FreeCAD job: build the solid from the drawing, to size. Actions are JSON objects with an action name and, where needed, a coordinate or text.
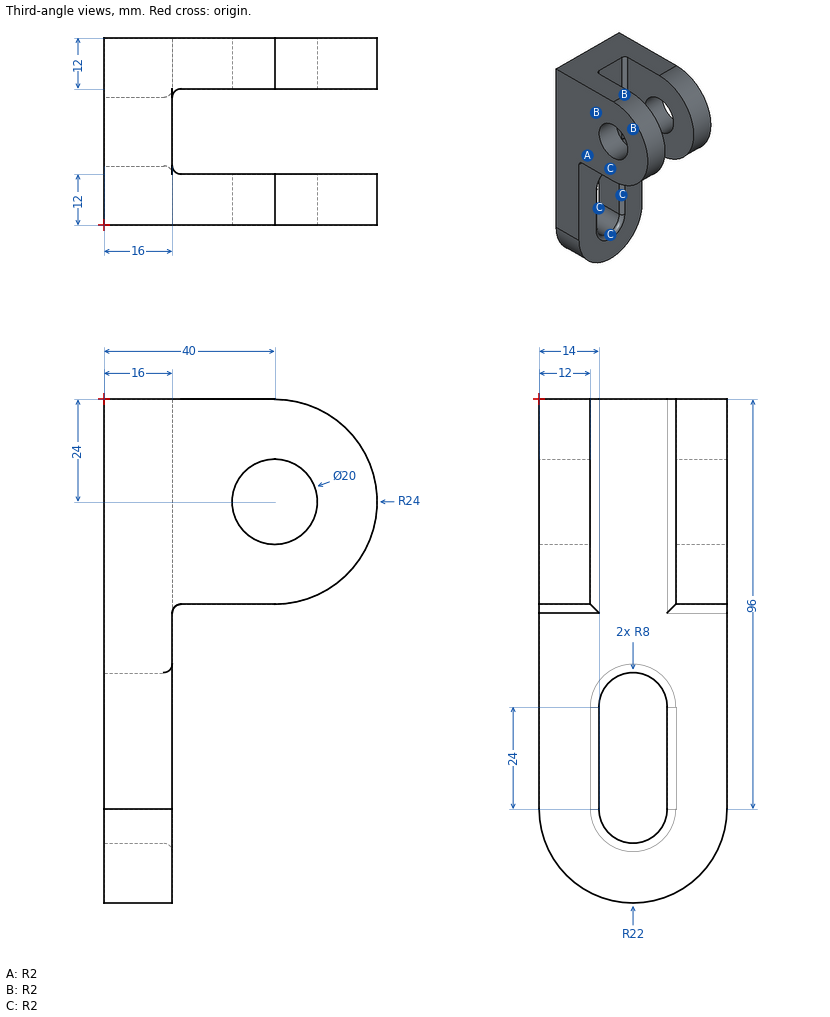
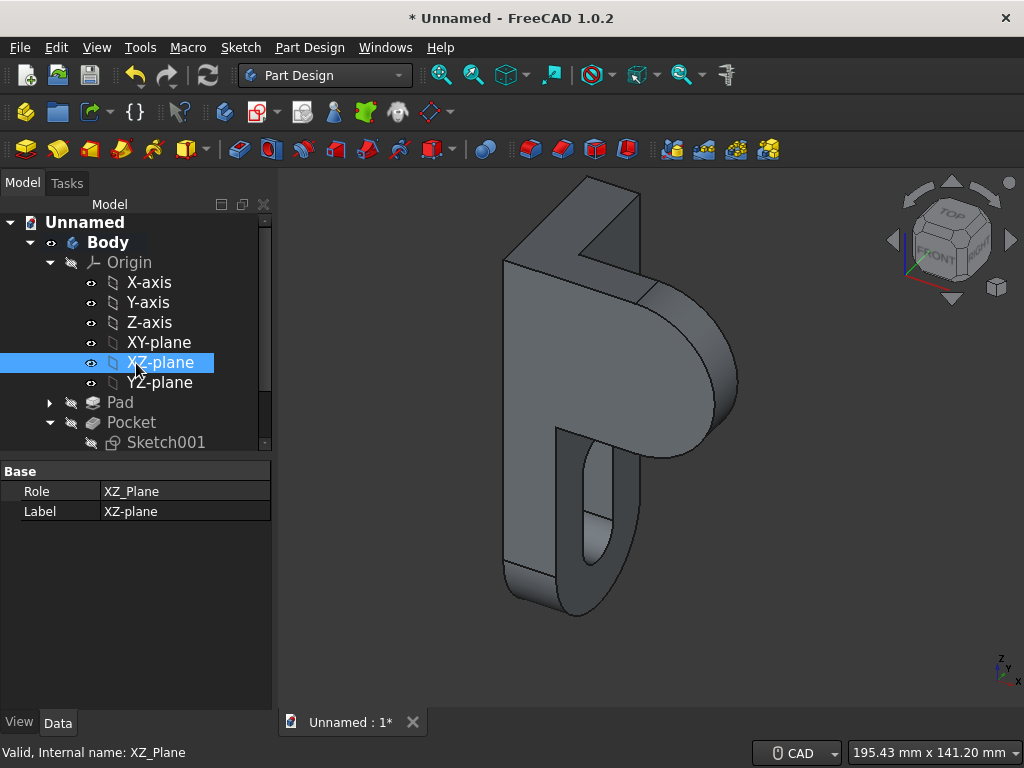
{"action": "left_click", "coordinate": [430, 112]}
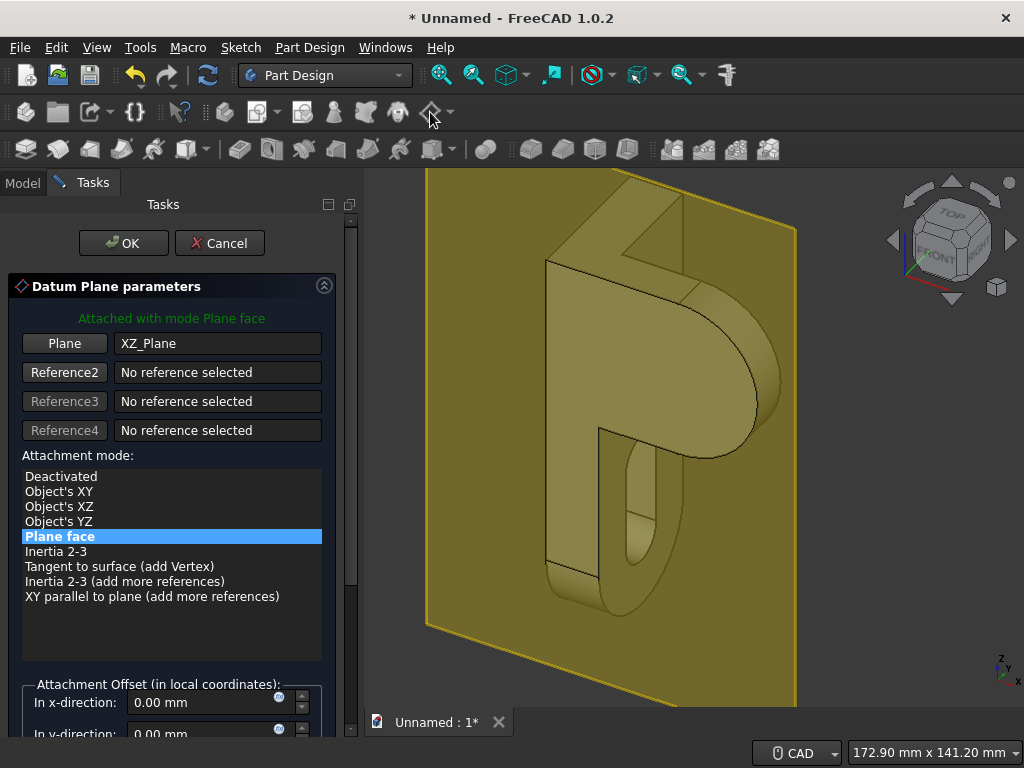
{"action": "scroll", "coordinate": [351, 475], "scroll_direction": "down", "scroll_amount": 2}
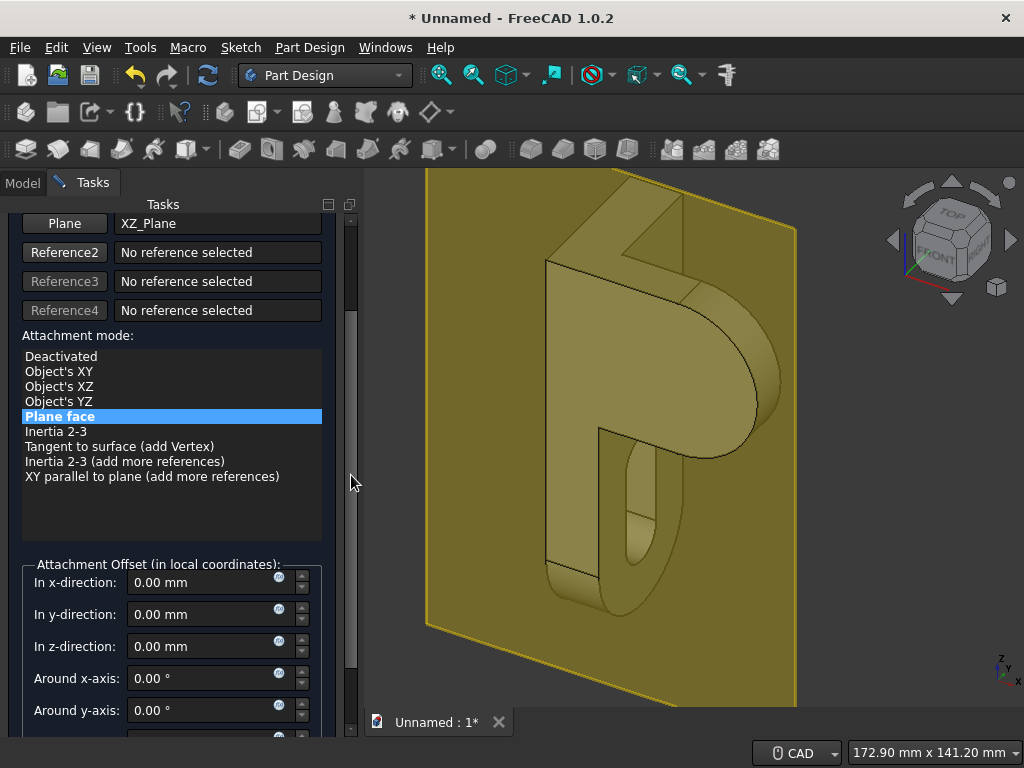
{"action": "triple_click", "coordinate": [210, 646]}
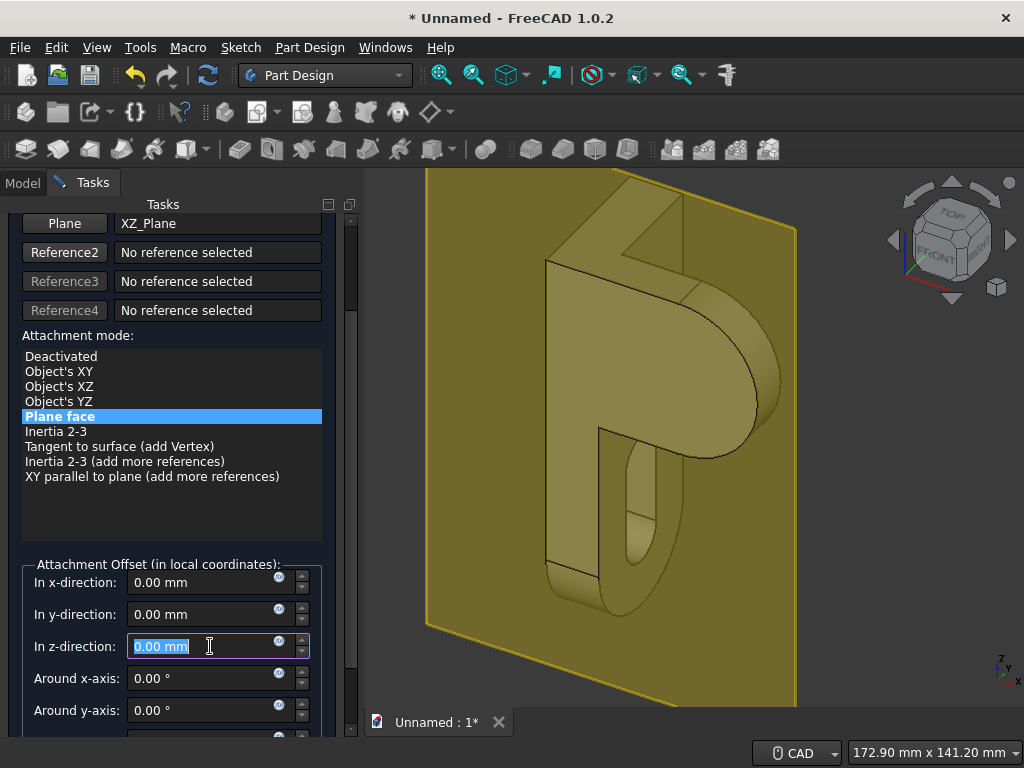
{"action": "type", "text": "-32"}
{"action": "key", "text": "Tab"}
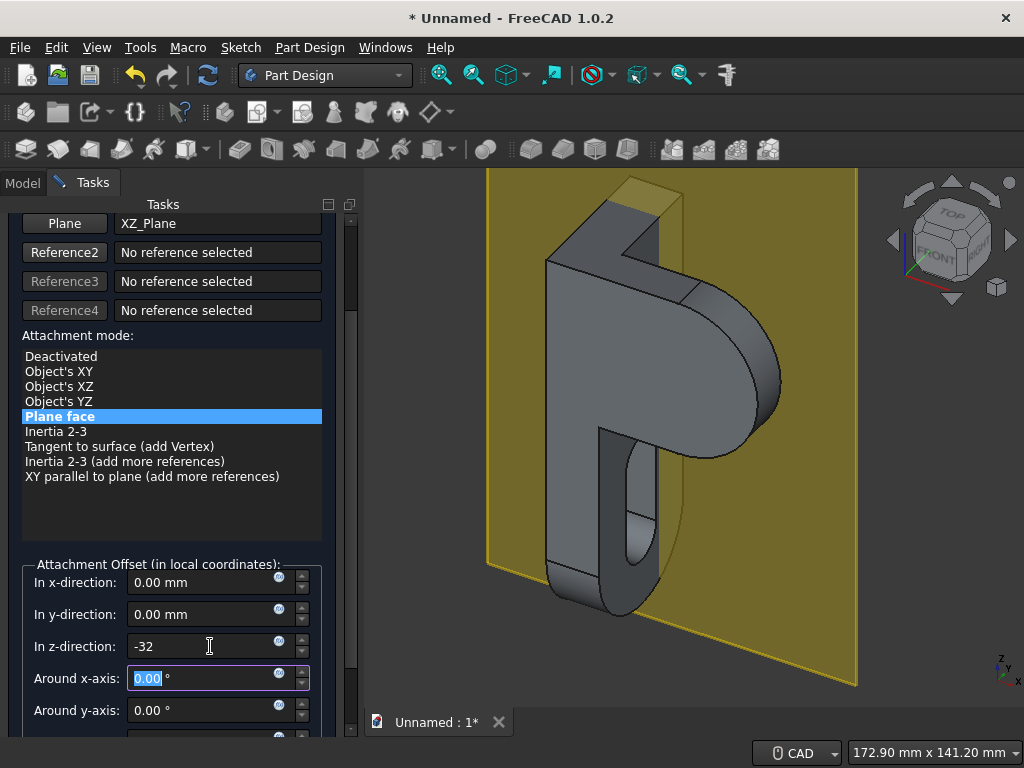
{"action": "scroll", "coordinate": [351, 475], "scroll_direction": "up", "scroll_amount": 3}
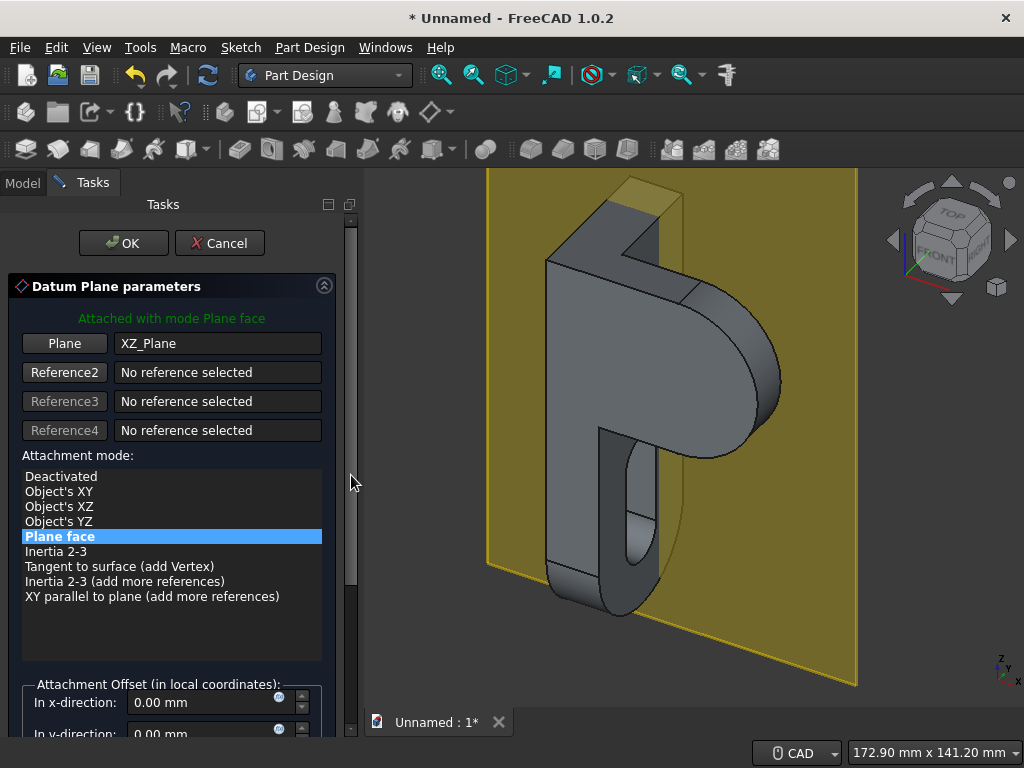
{"action": "left_click", "coordinate": [124, 243]}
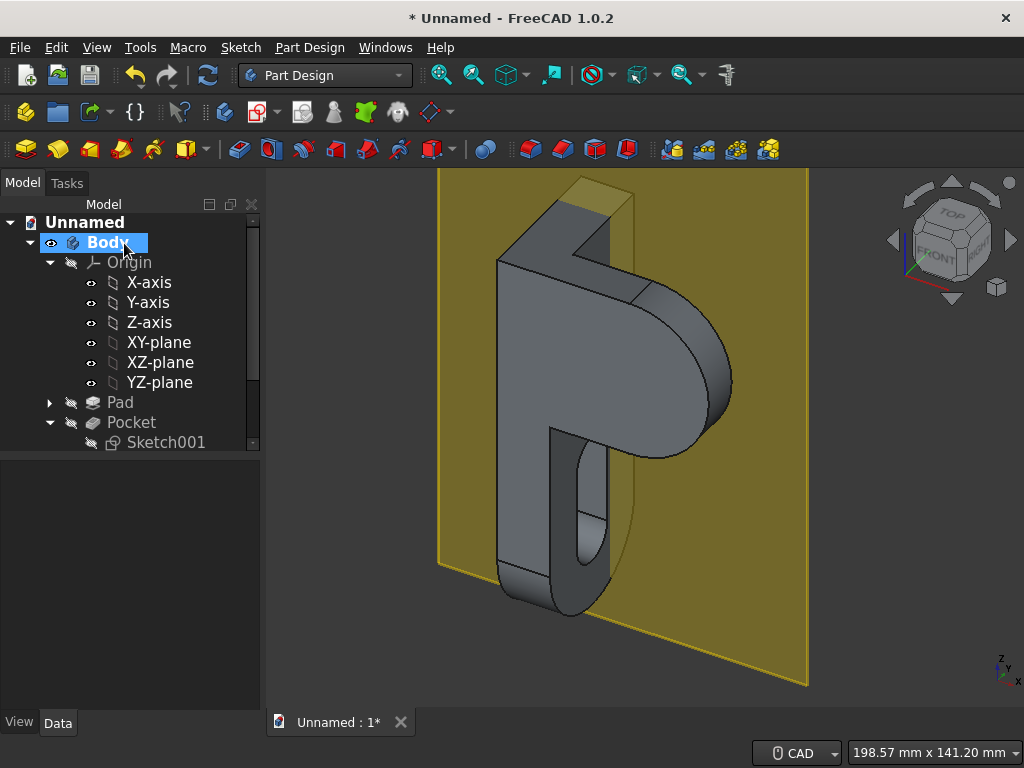
{"action": "scroll", "coordinate": [100, 338], "scroll_direction": "down", "scroll_amount": 3}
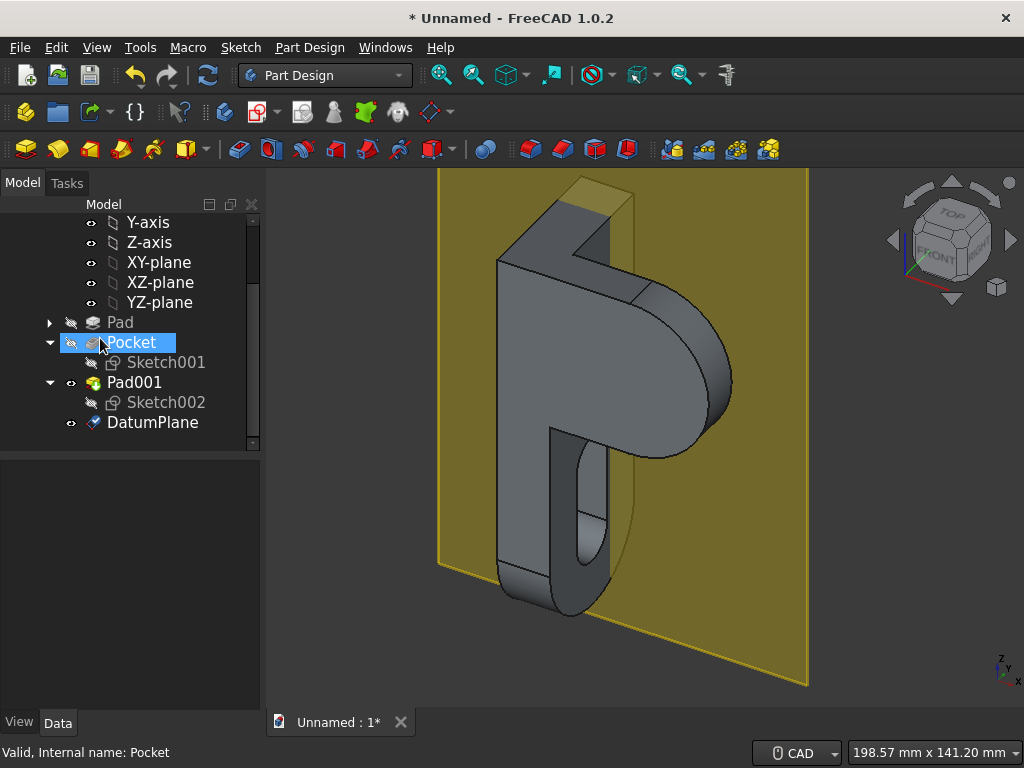
{"action": "left_click", "coordinate": [116, 423]}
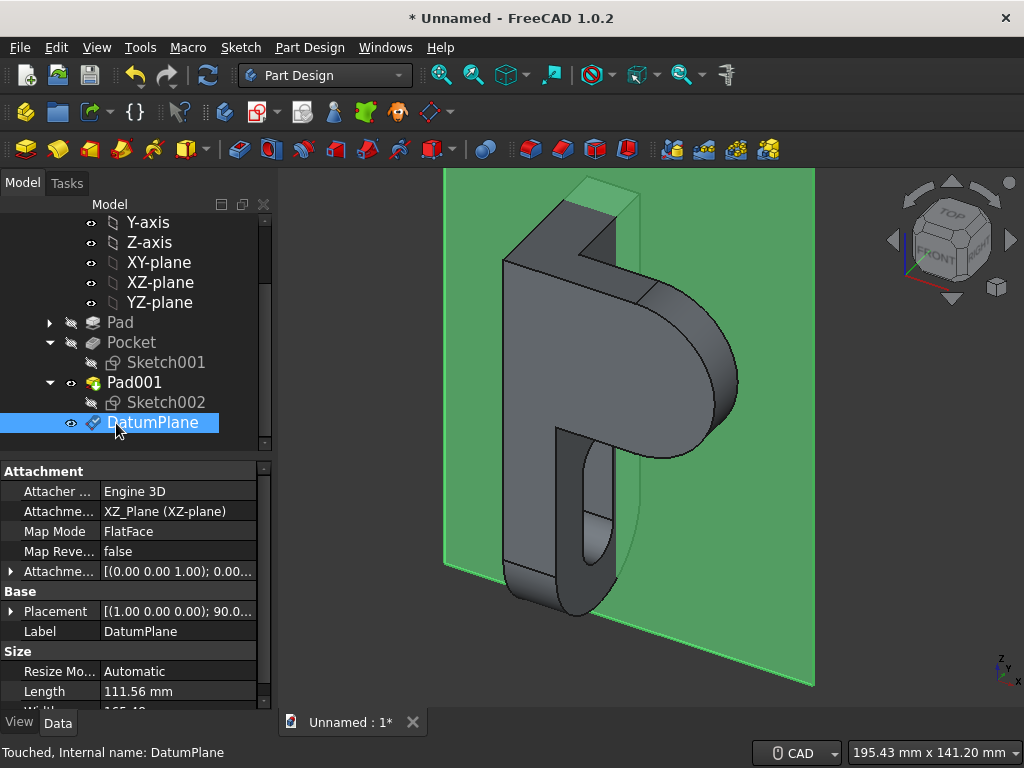
{"action": "left_click", "coordinate": [258, 112]}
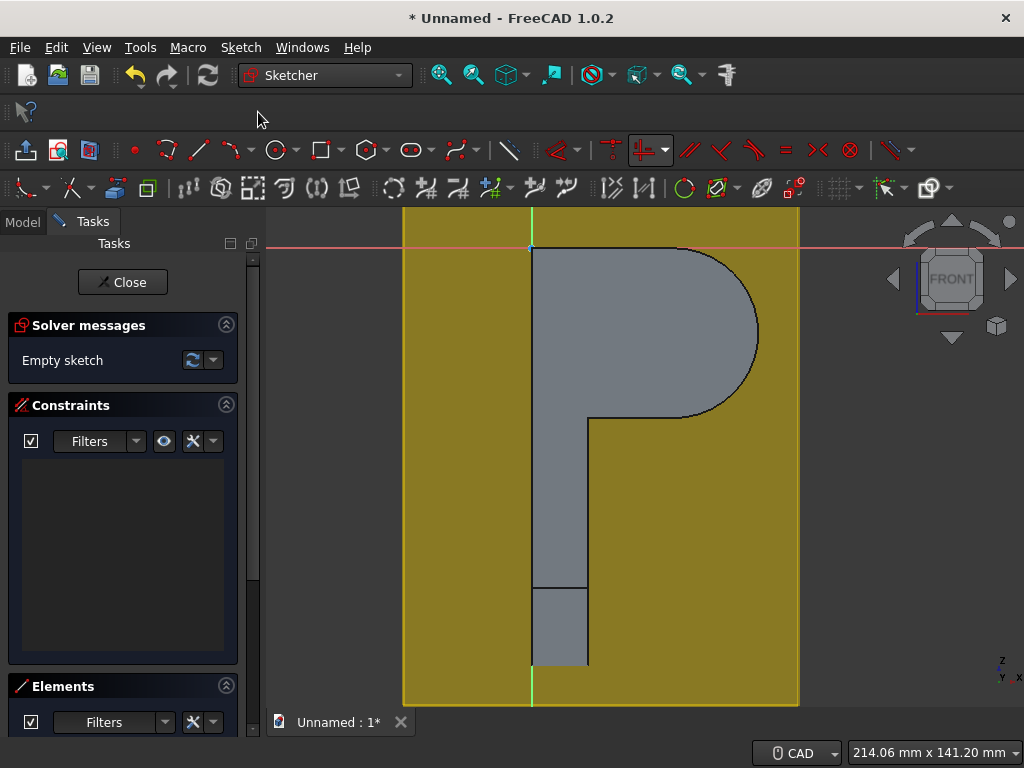
{"action": "left_click", "coordinate": [90, 150]}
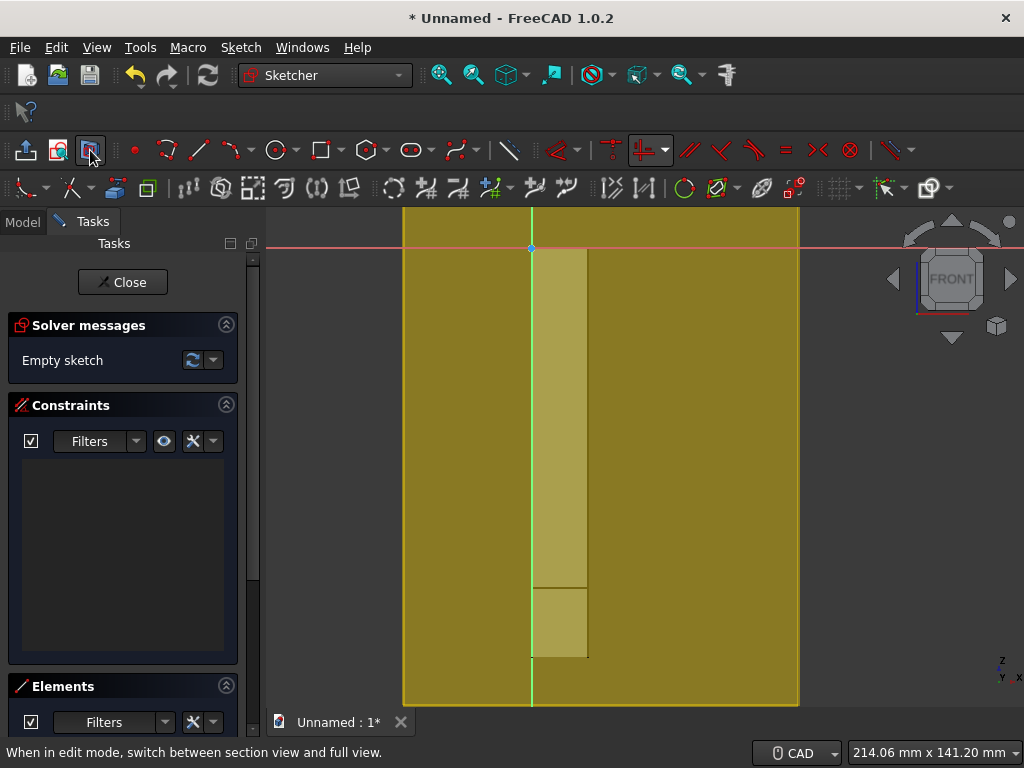
{"action": "scroll", "coordinate": [576, 457], "scroll_direction": "down", "scroll_amount": 5}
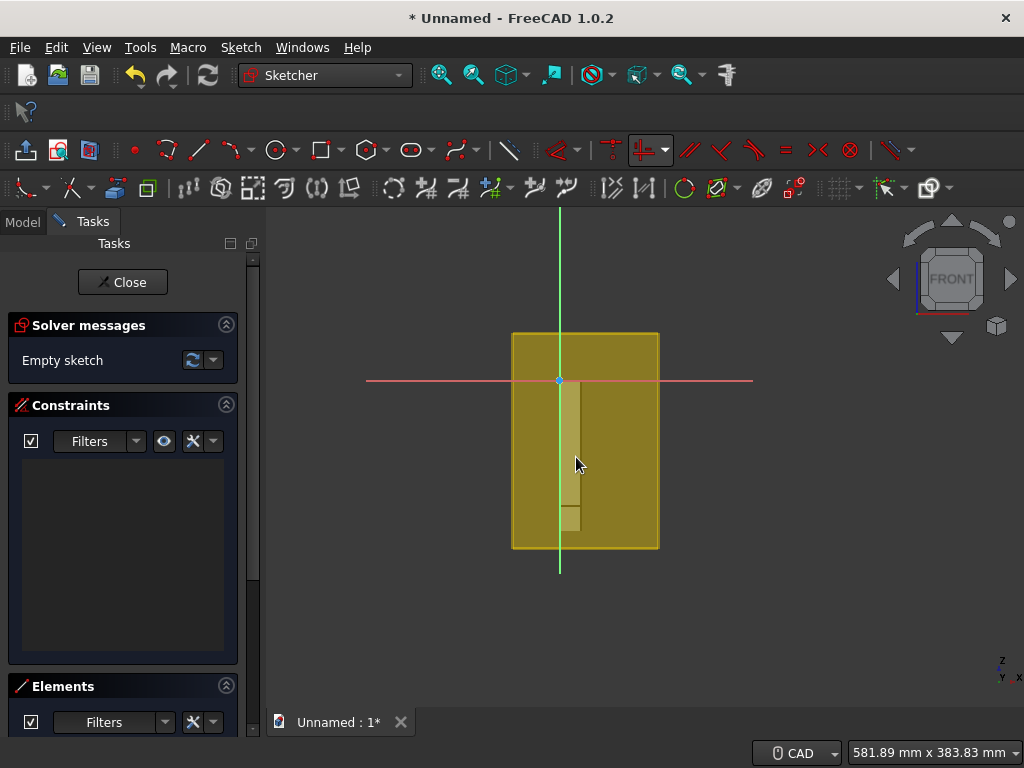
{"action": "scroll", "coordinate": [608, 400], "scroll_direction": "up", "scroll_amount": 8}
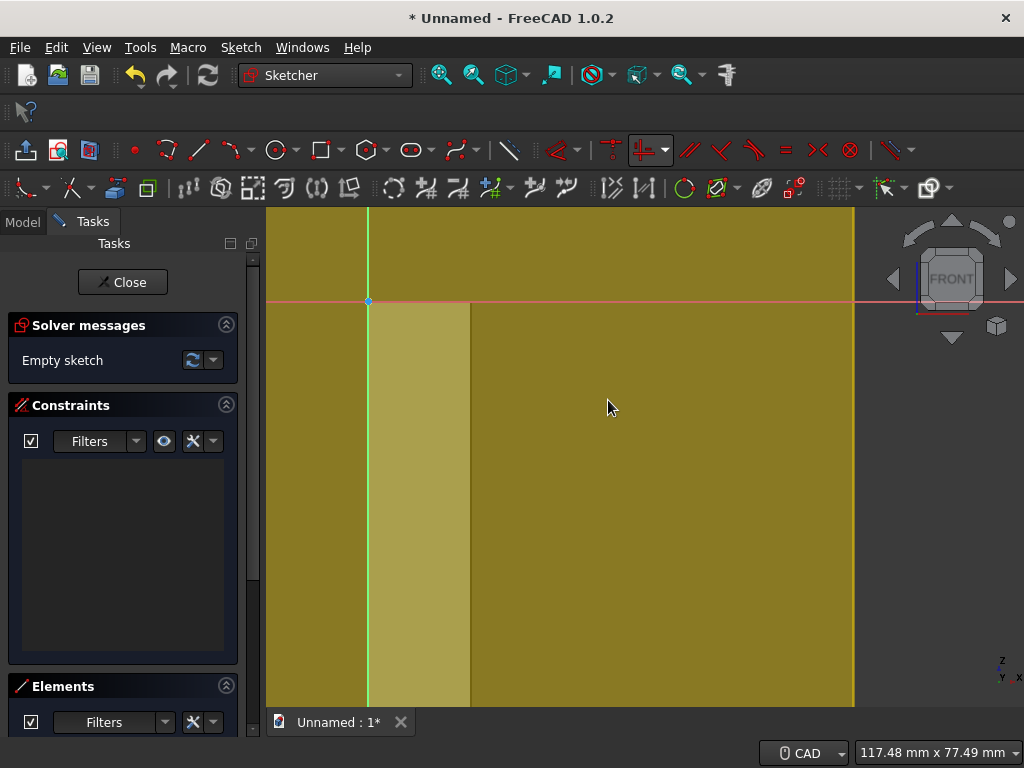
{"action": "left_click", "coordinate": [168, 150]}